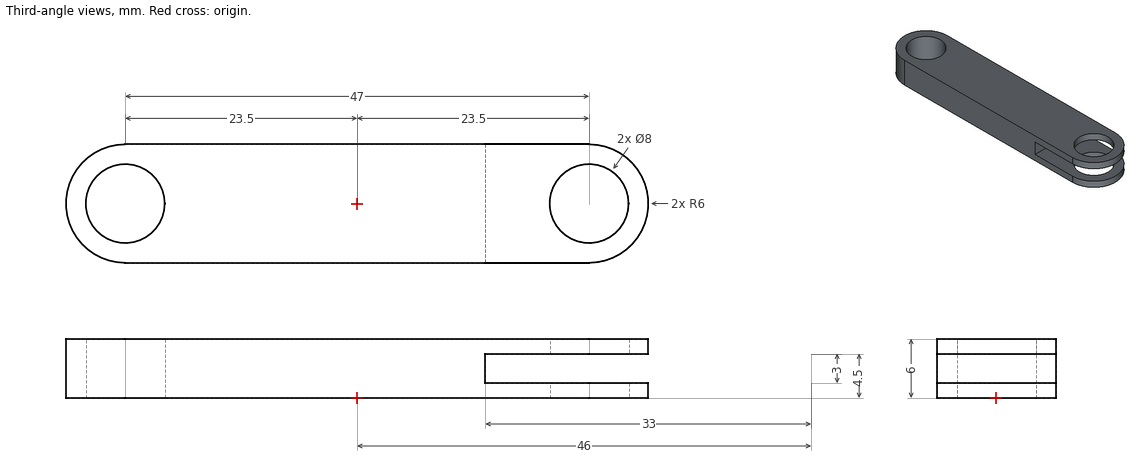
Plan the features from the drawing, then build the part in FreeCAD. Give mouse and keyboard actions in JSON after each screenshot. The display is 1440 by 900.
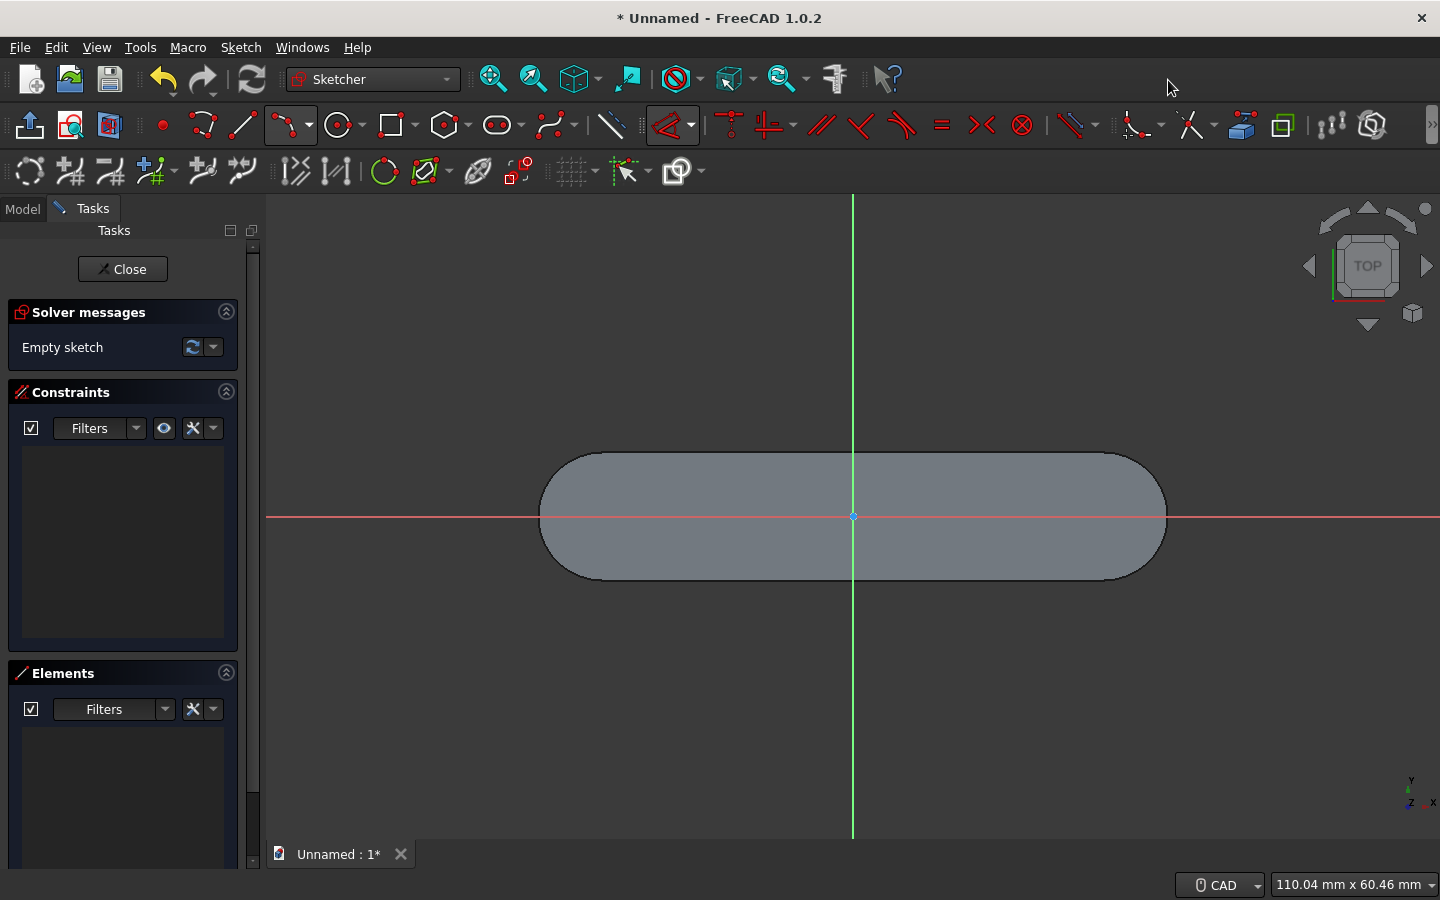
{"action": "key", "text": "g c"}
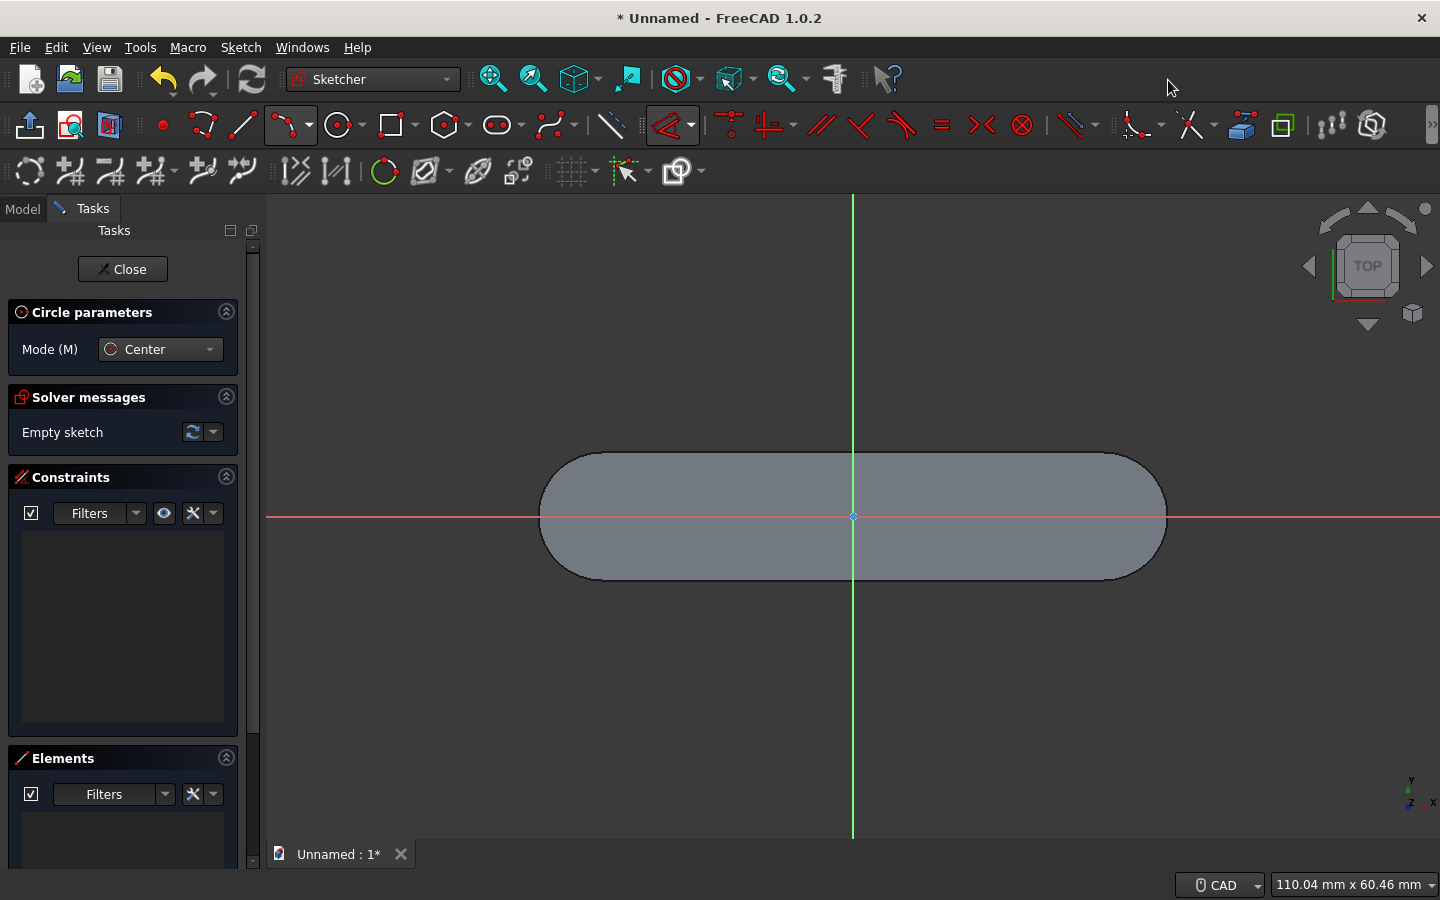
{"action": "left_click", "coordinate": [1104, 516]}
{"action": "left_click", "coordinate": [1134, 486]}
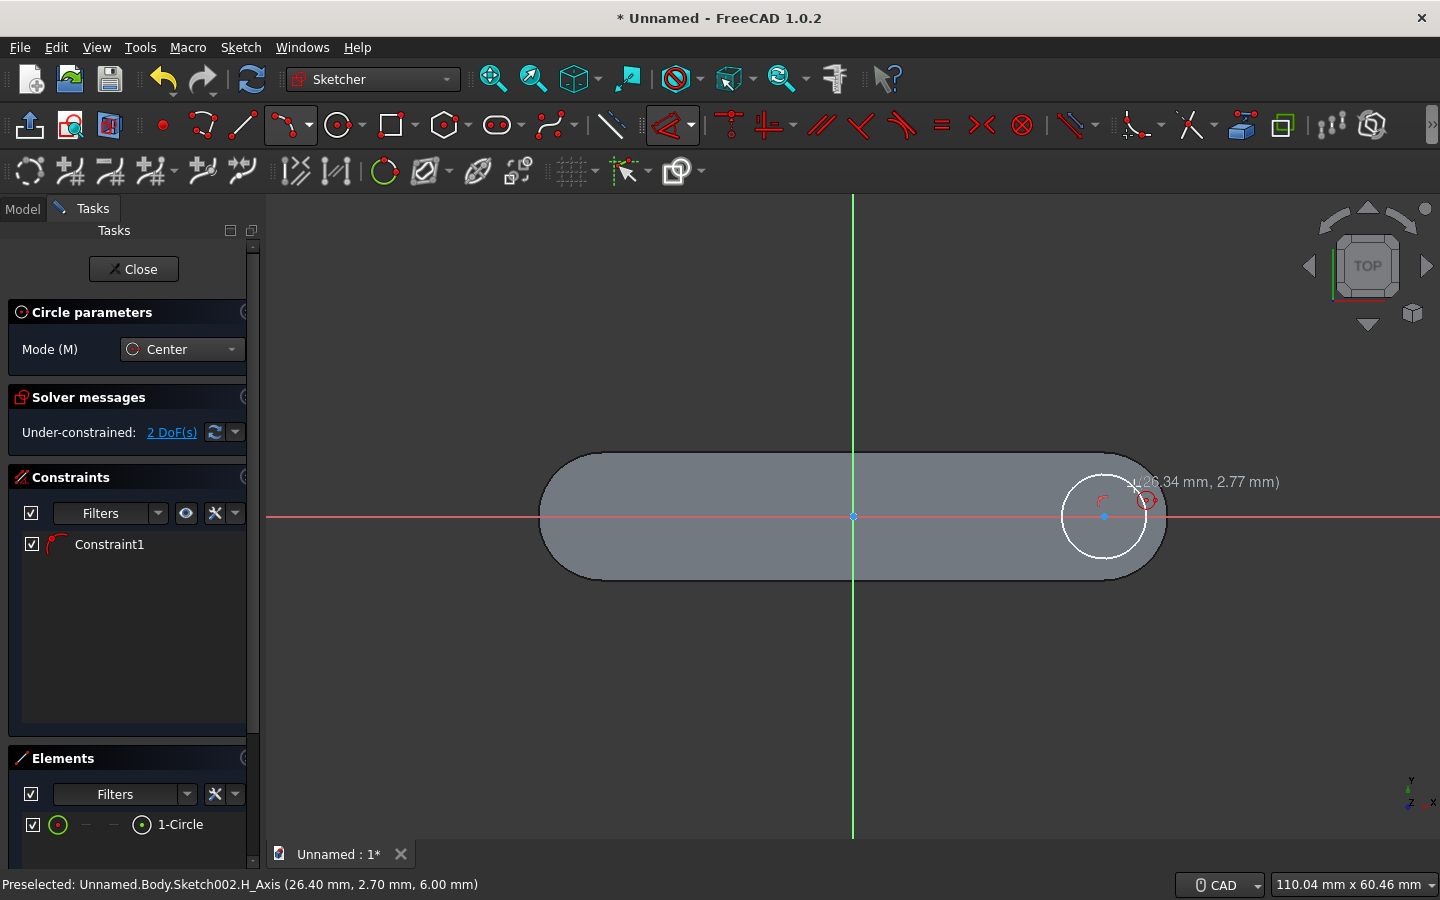
{"action": "left_click", "coordinate": [602, 516]}
{"action": "left_click", "coordinate": [632, 486]}
{"action": "key", "text": "Escape"}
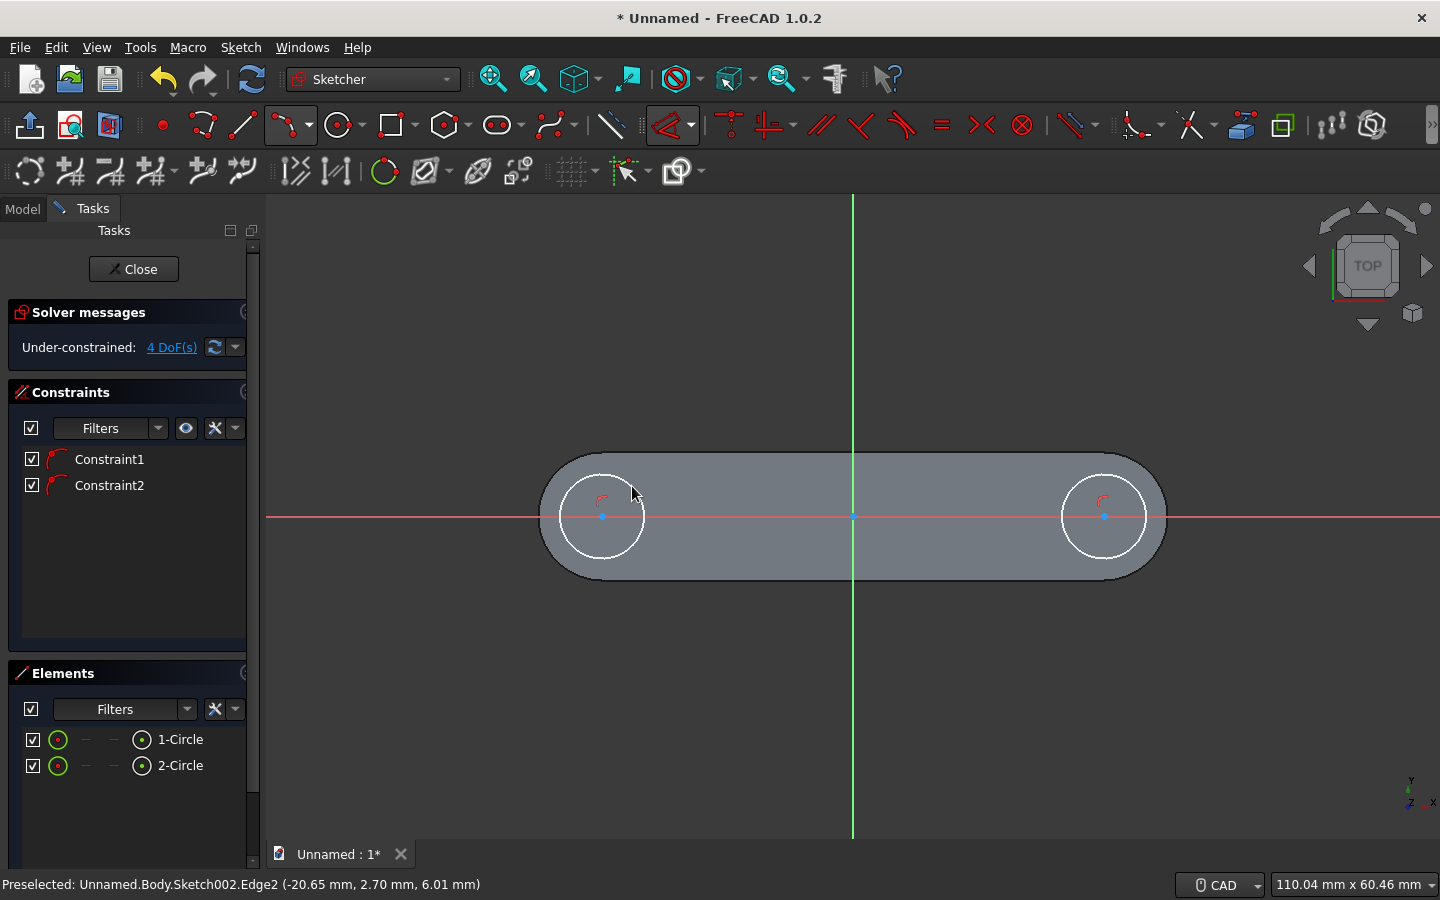
{"action": "left_click", "coordinate": [1134, 487]}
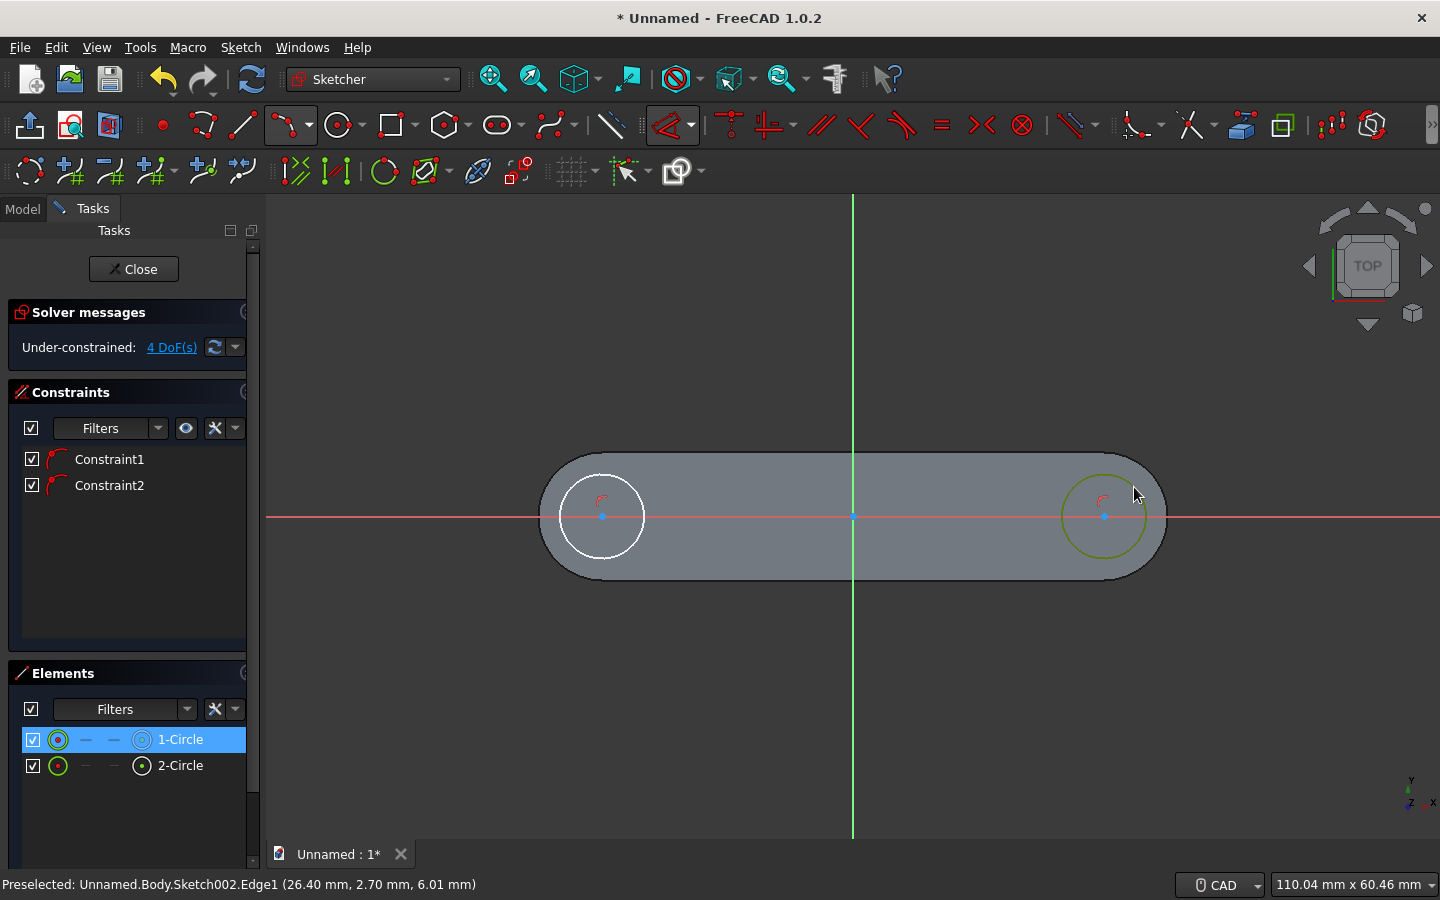
{"action": "left_click", "coordinate": [632, 487]}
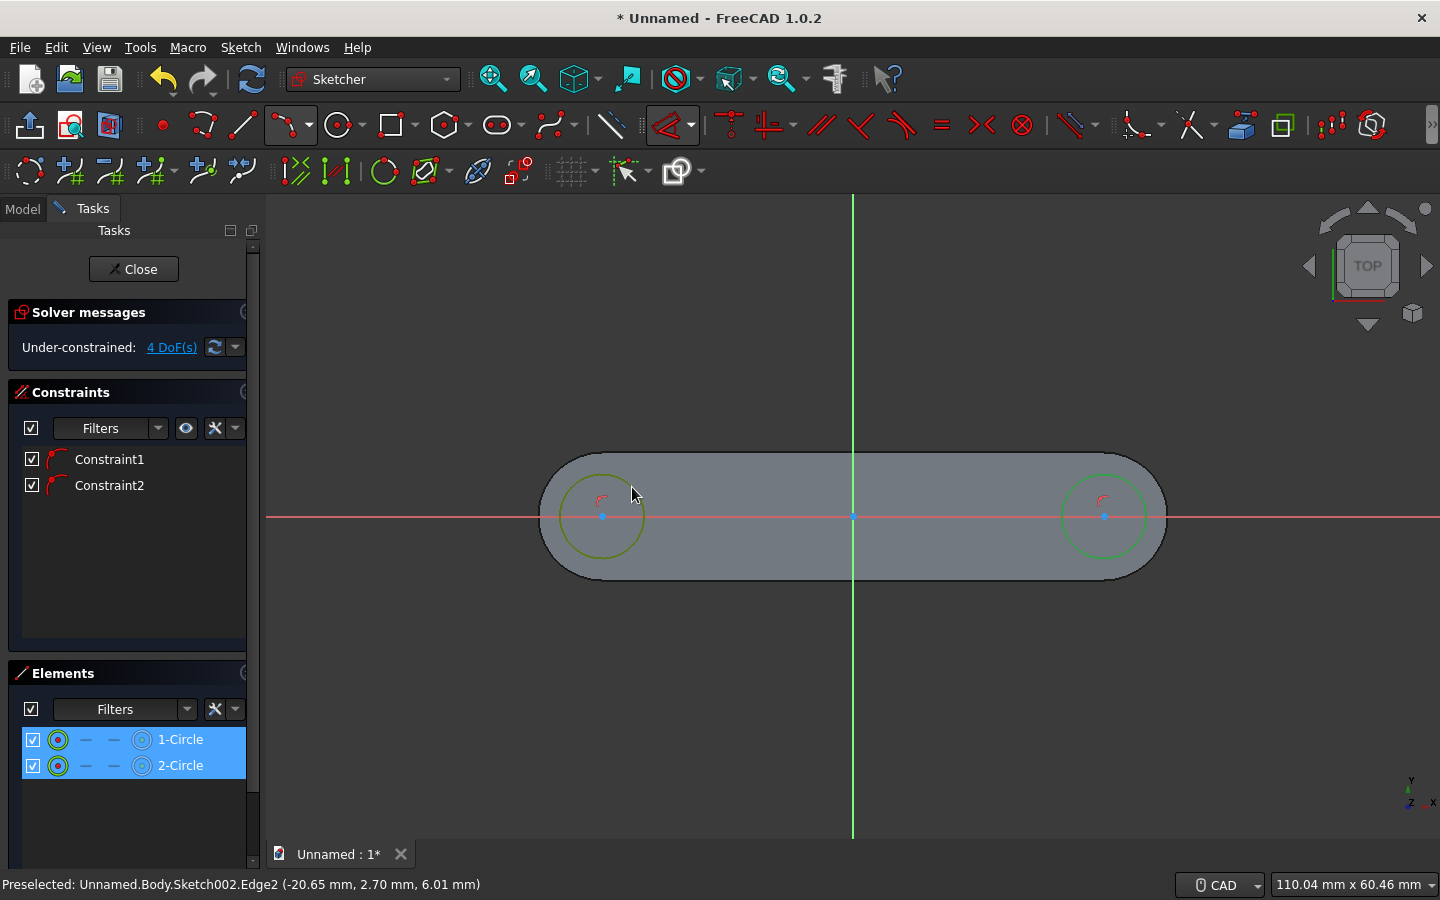
{"action": "left_click", "coordinate": [942, 126]}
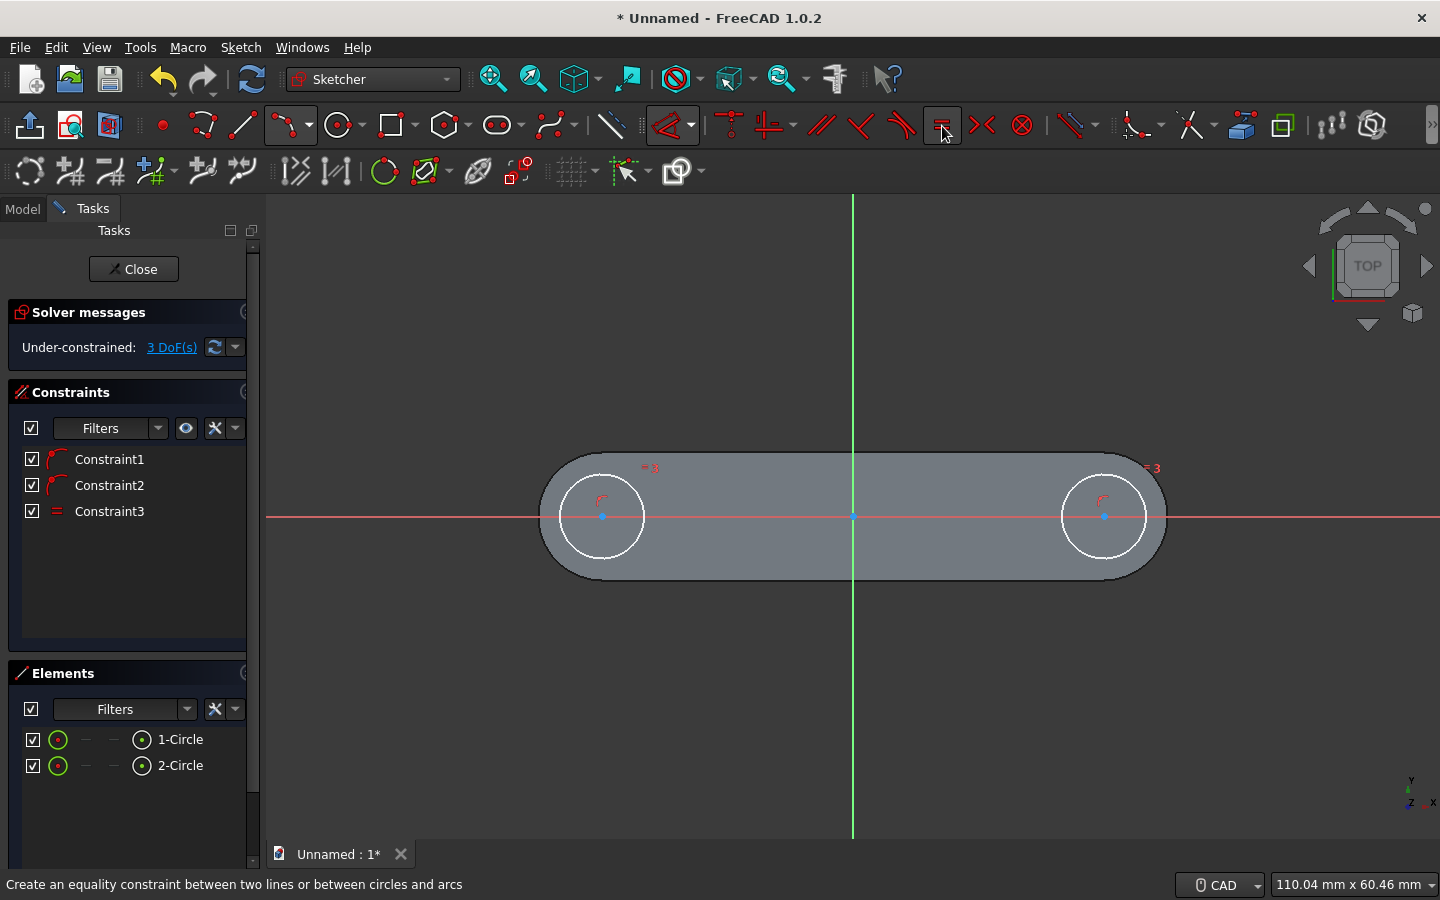
{"action": "left_click", "coordinate": [1134, 487]}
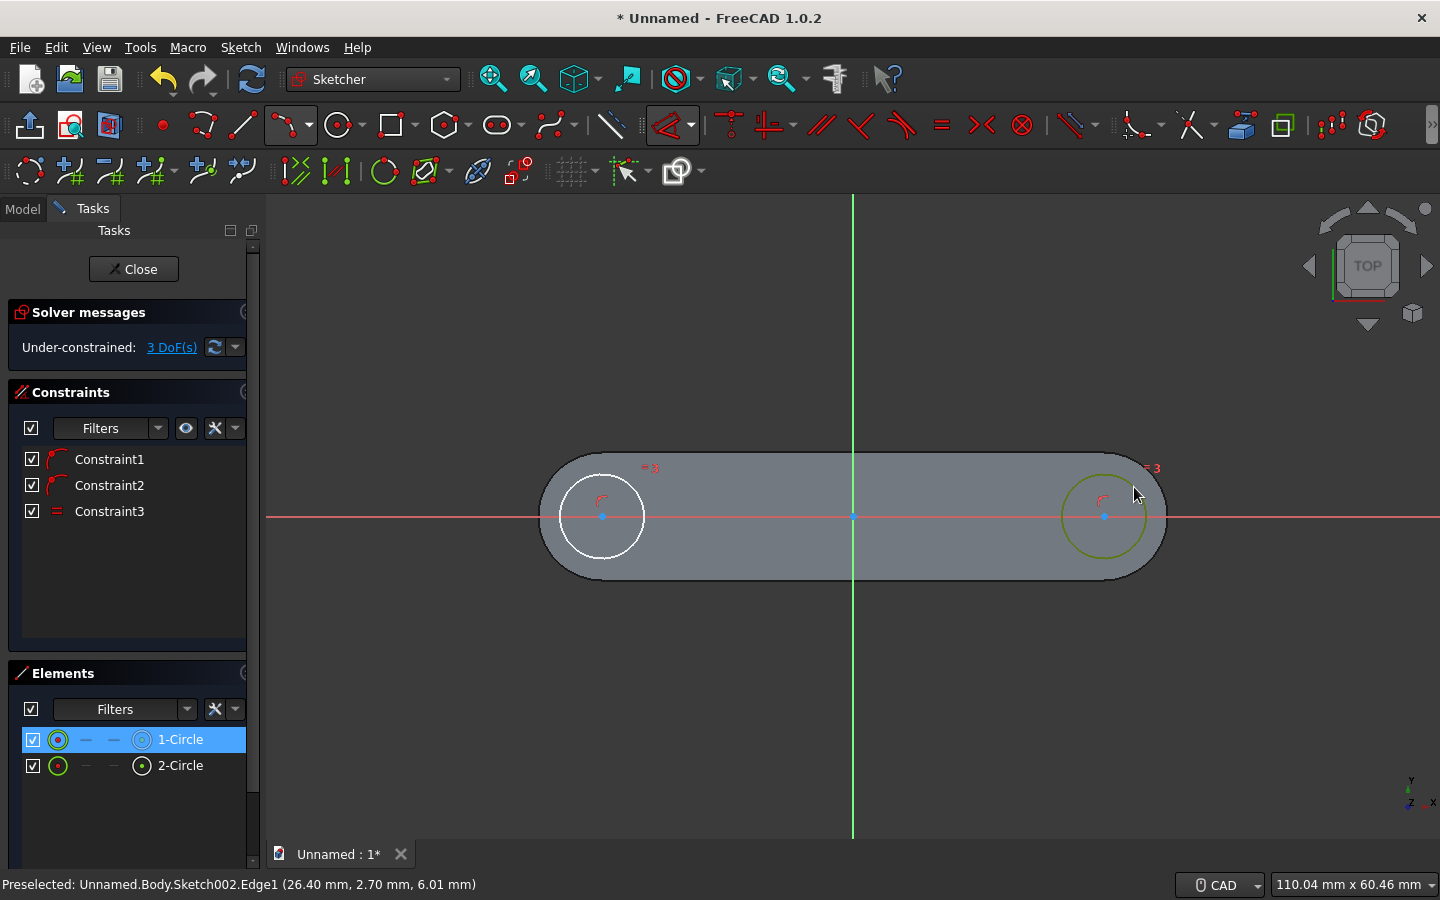
{"action": "key", "text": "k o"}